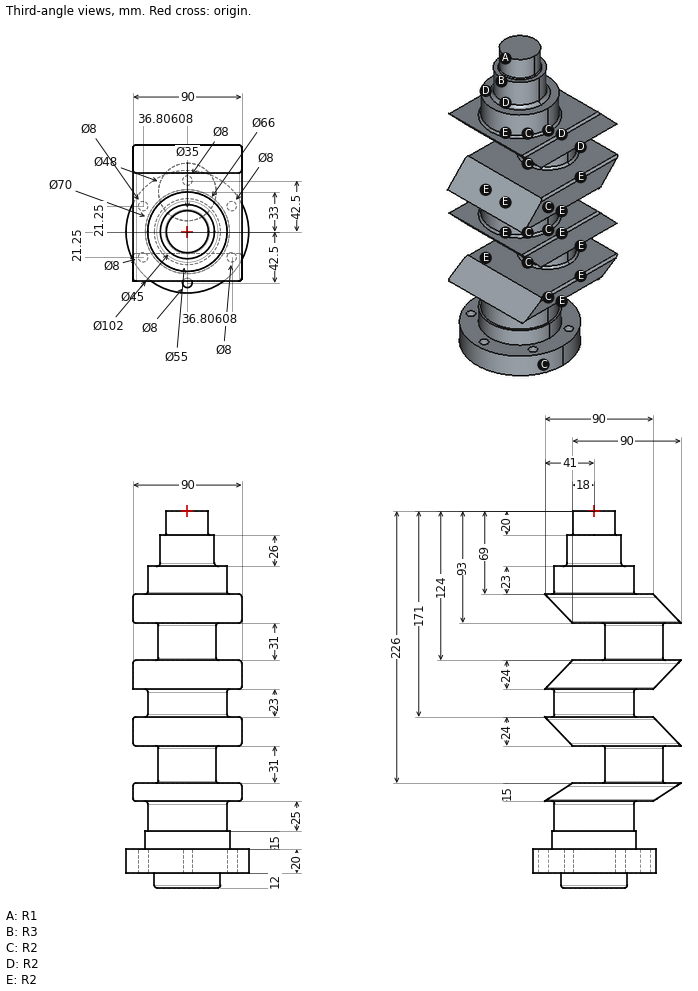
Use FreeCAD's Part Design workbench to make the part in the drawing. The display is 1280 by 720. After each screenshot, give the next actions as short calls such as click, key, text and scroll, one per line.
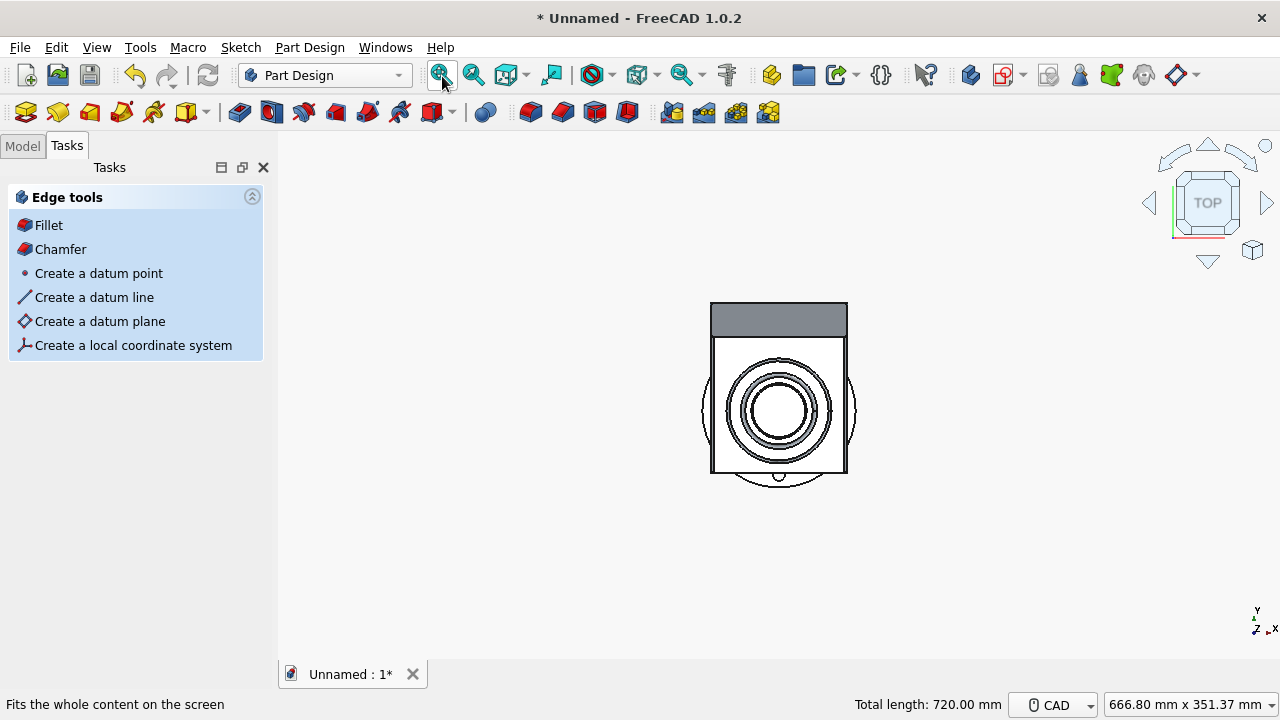
key(1)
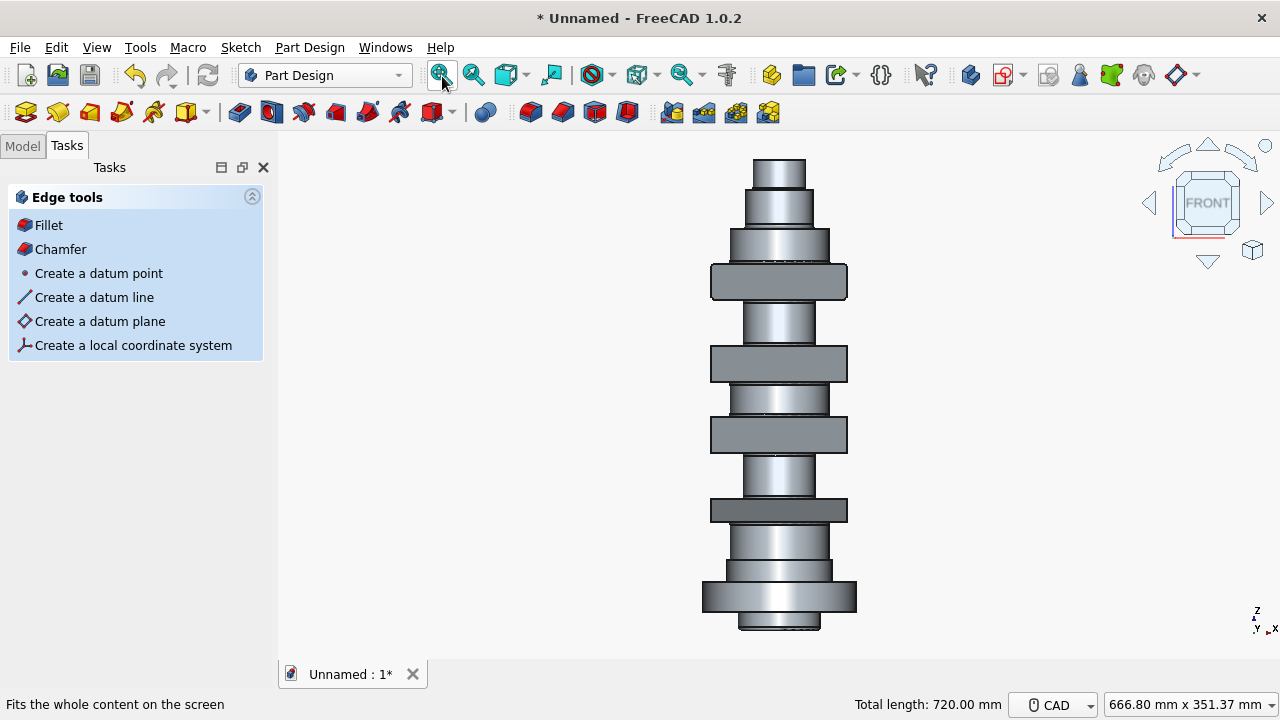
key(3)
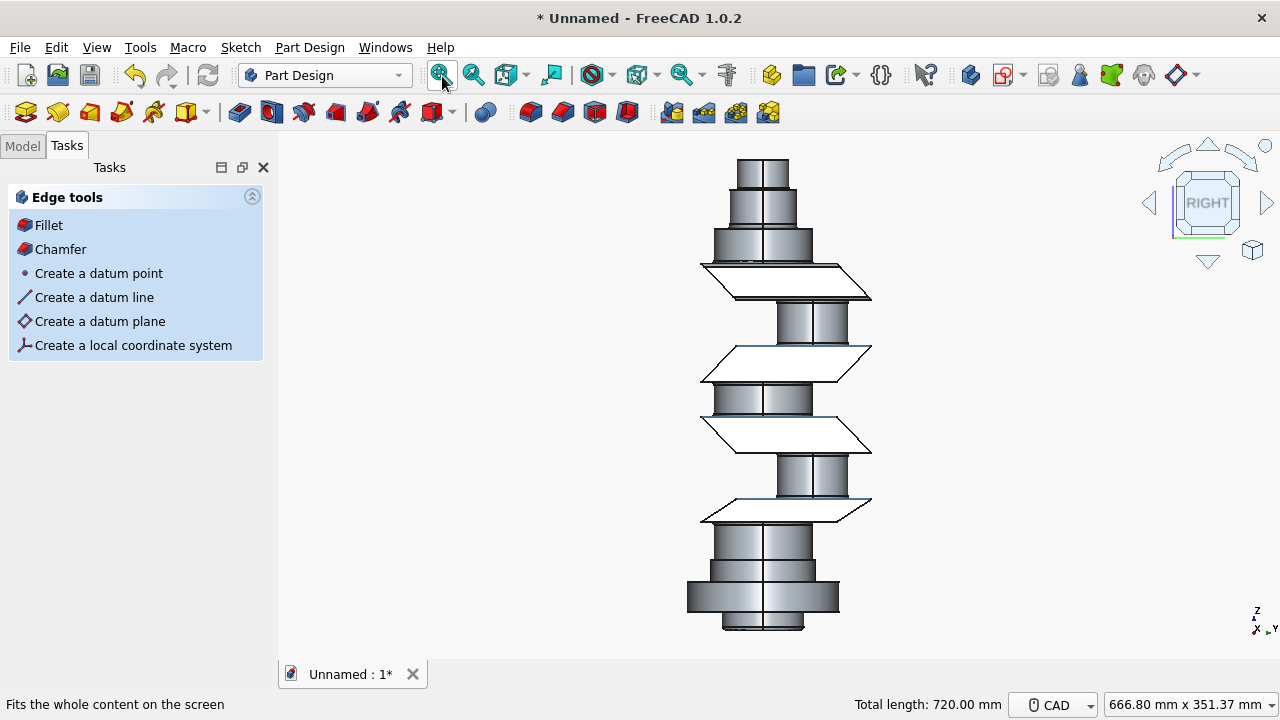
click(769, 381, ctrl)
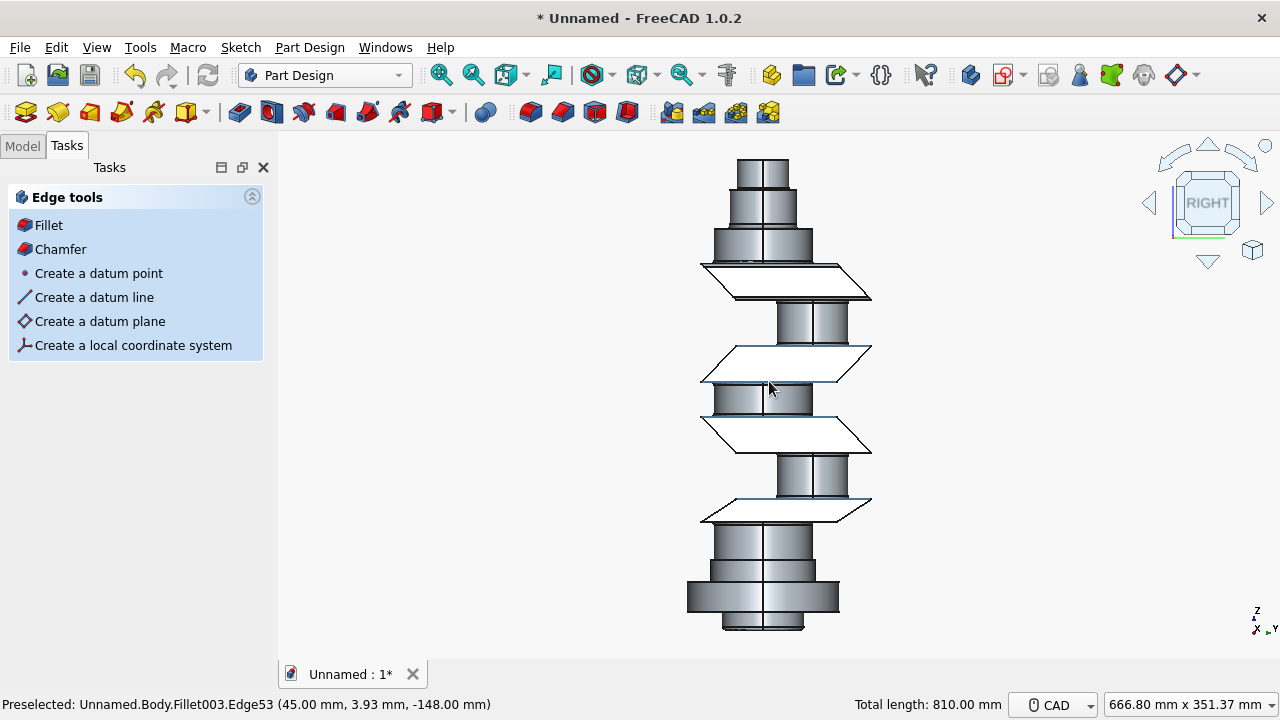
click(804, 452, ctrl)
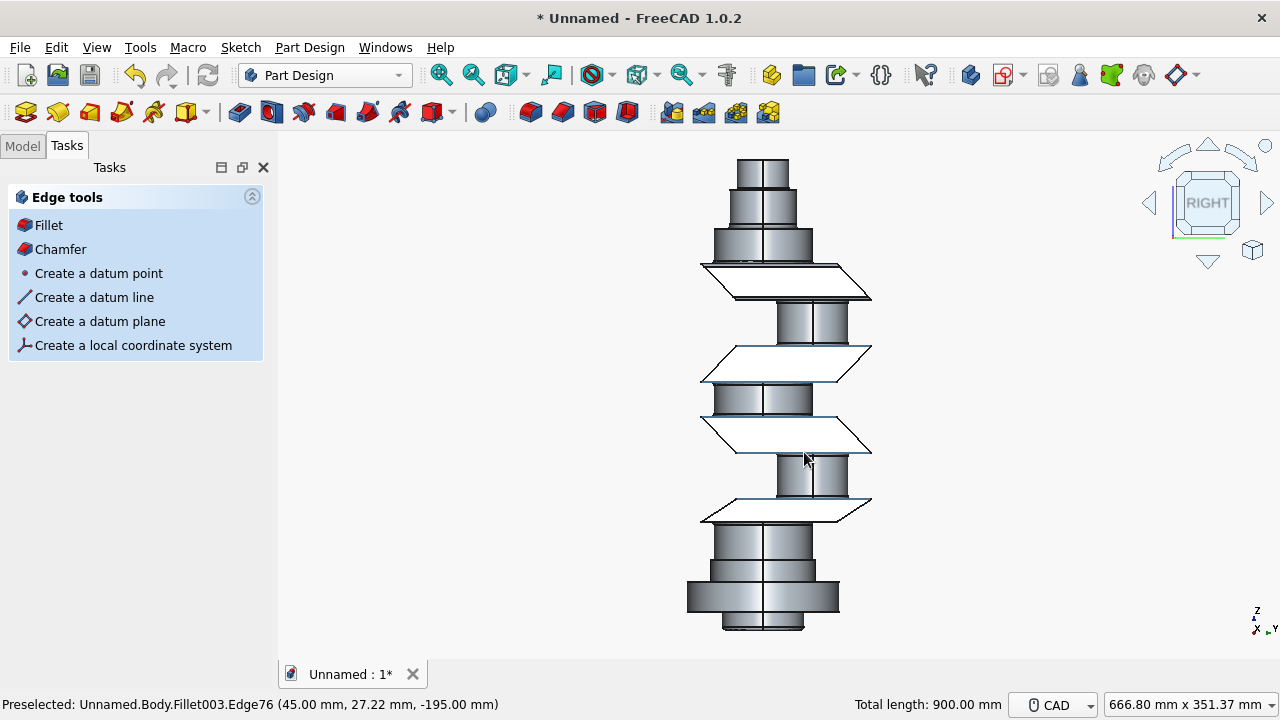
click(769, 521, ctrl)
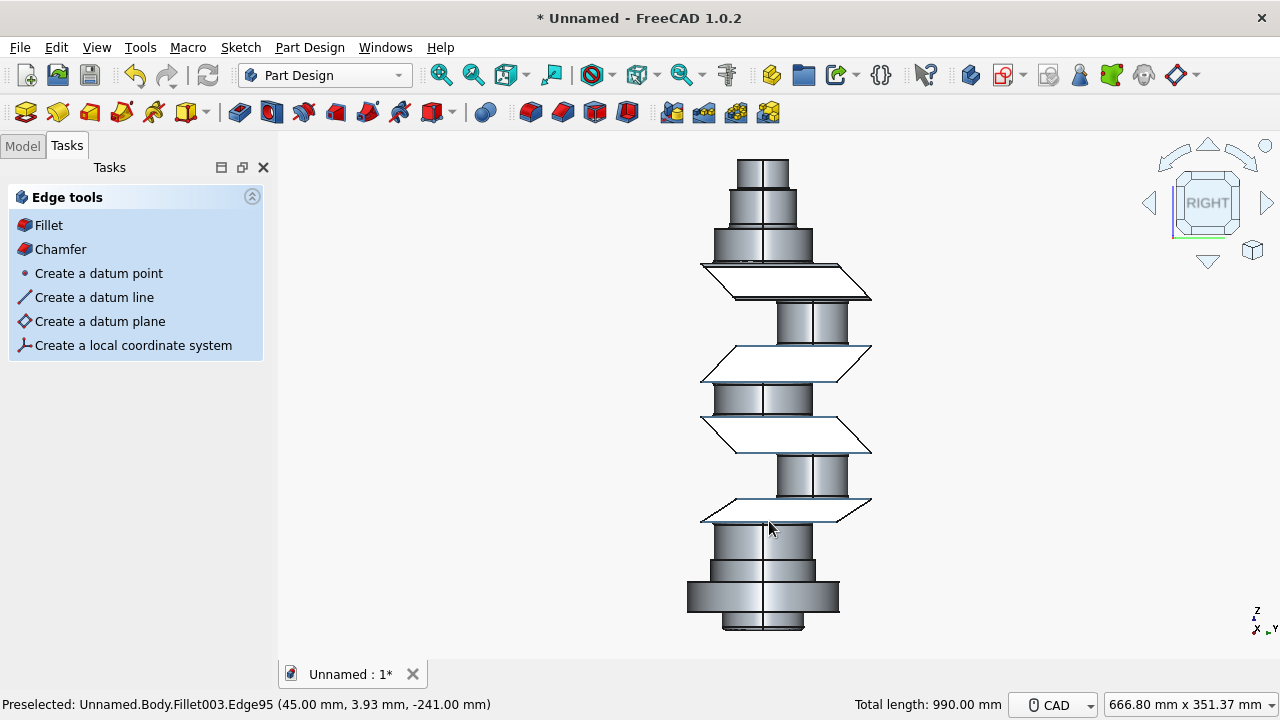
click(532, 112)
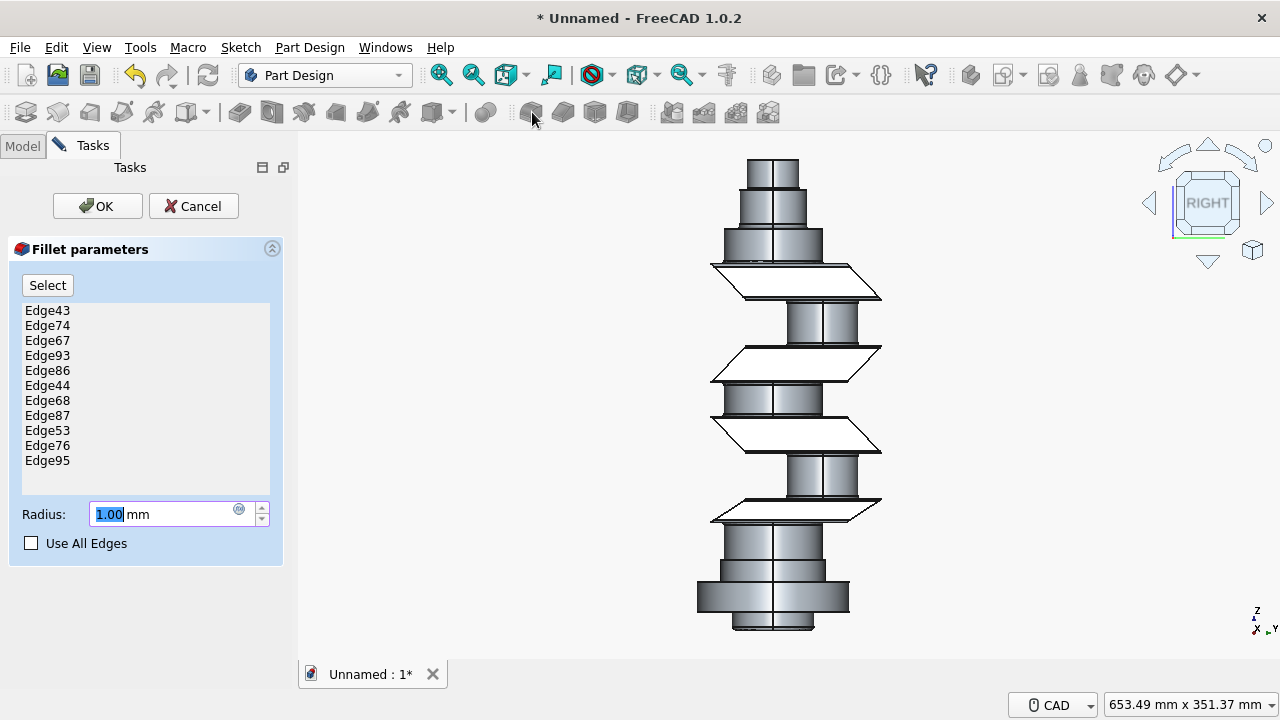
text(2)
key(Tab)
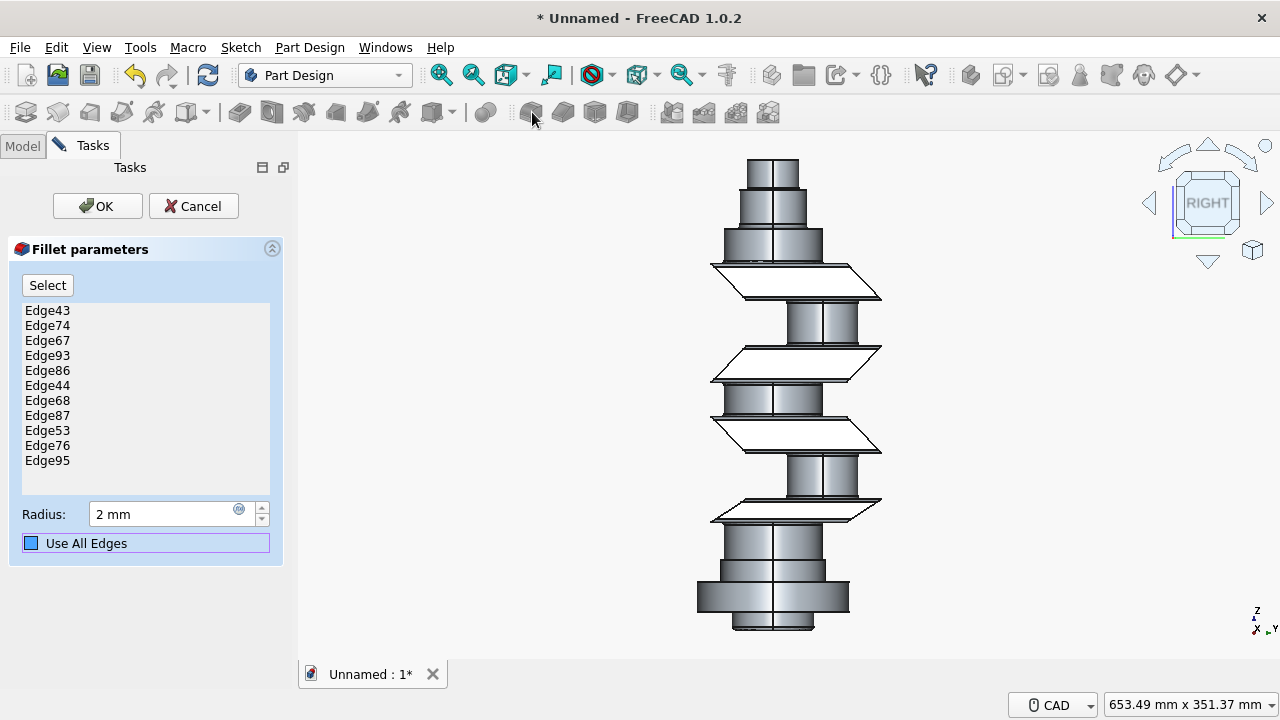
click(98, 206)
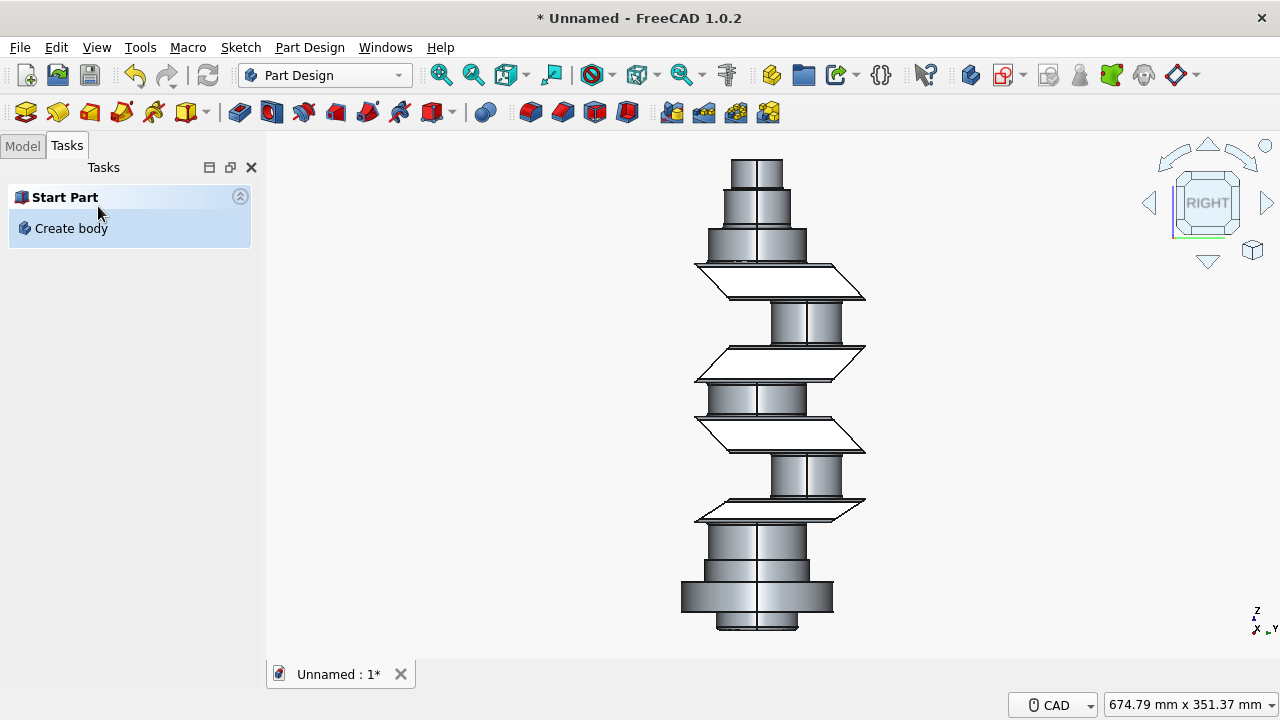
key(0)